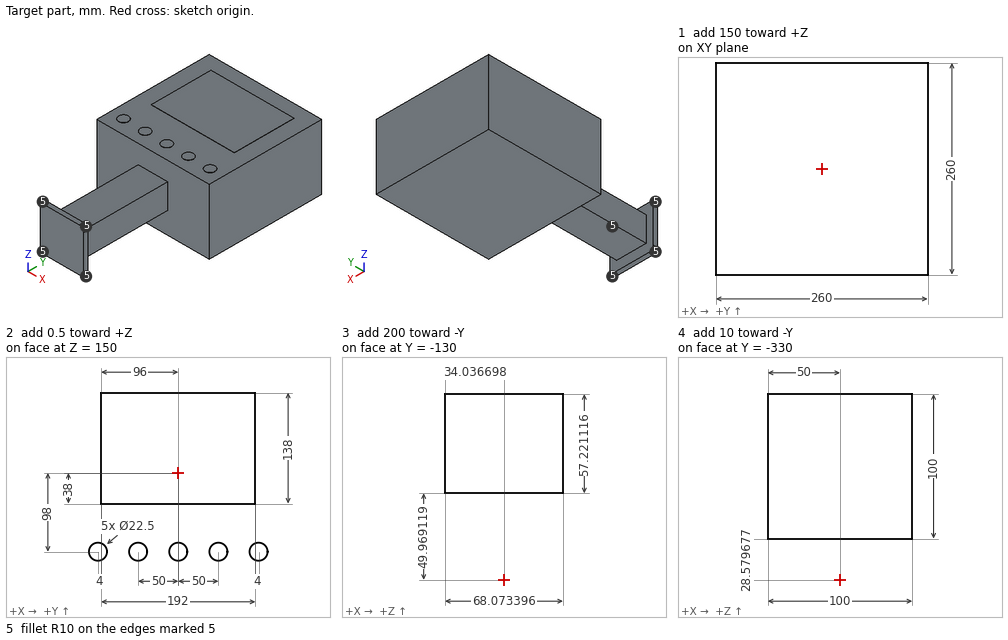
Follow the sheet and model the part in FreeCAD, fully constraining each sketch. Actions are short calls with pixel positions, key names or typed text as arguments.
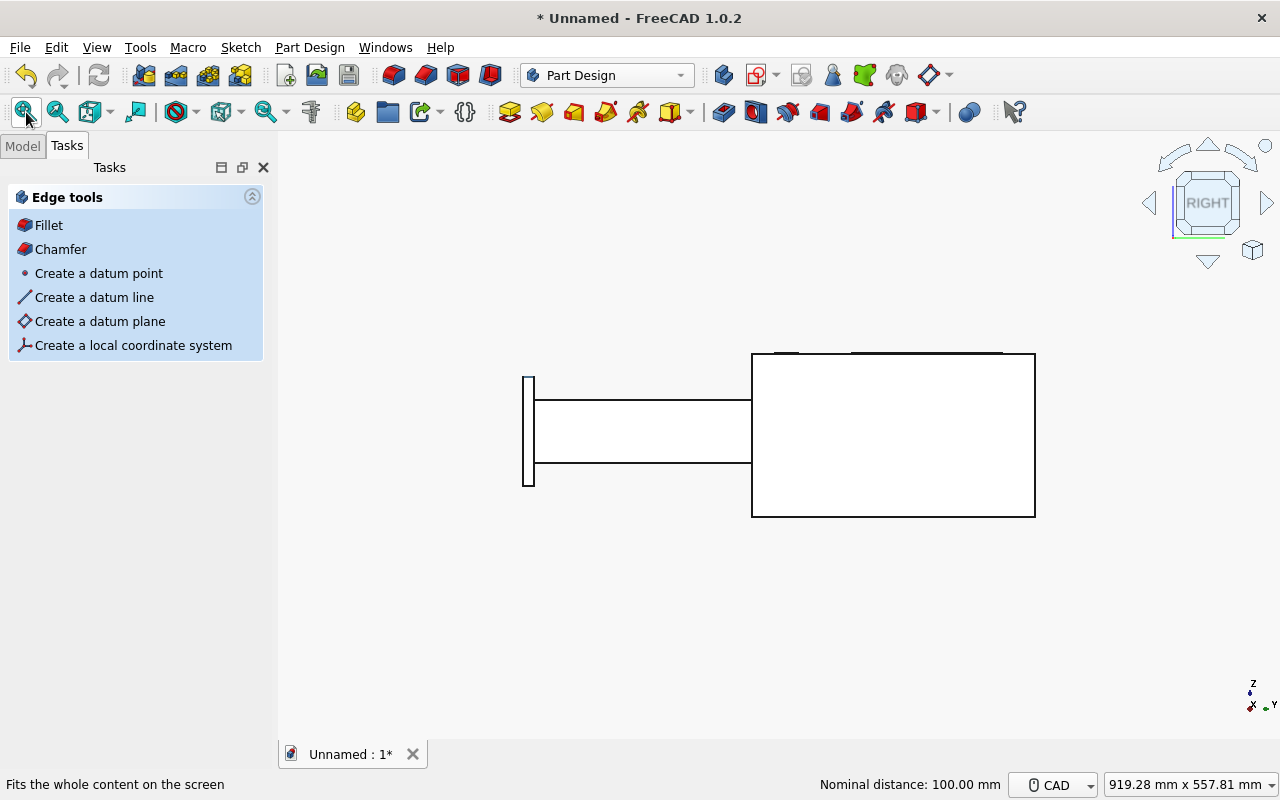
scroll(528, 485, up, 7)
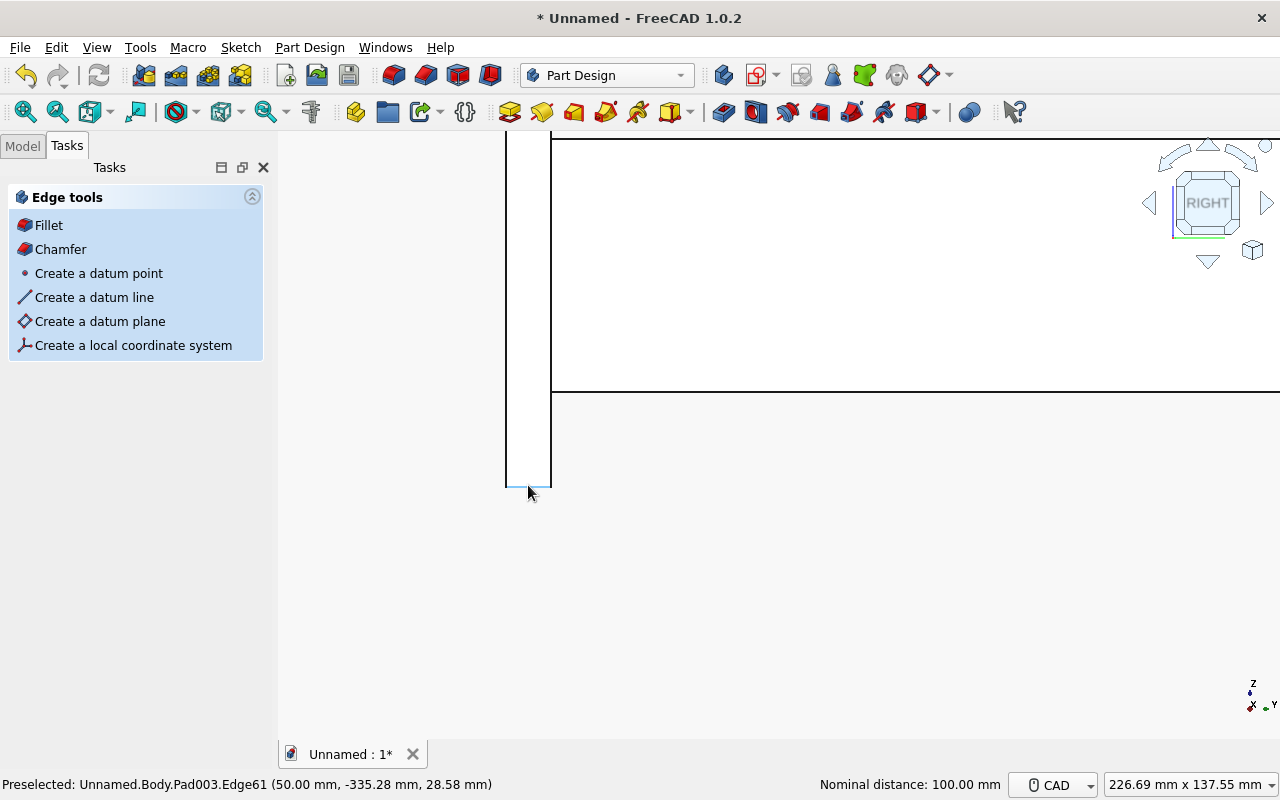
click(528, 486, ctrl)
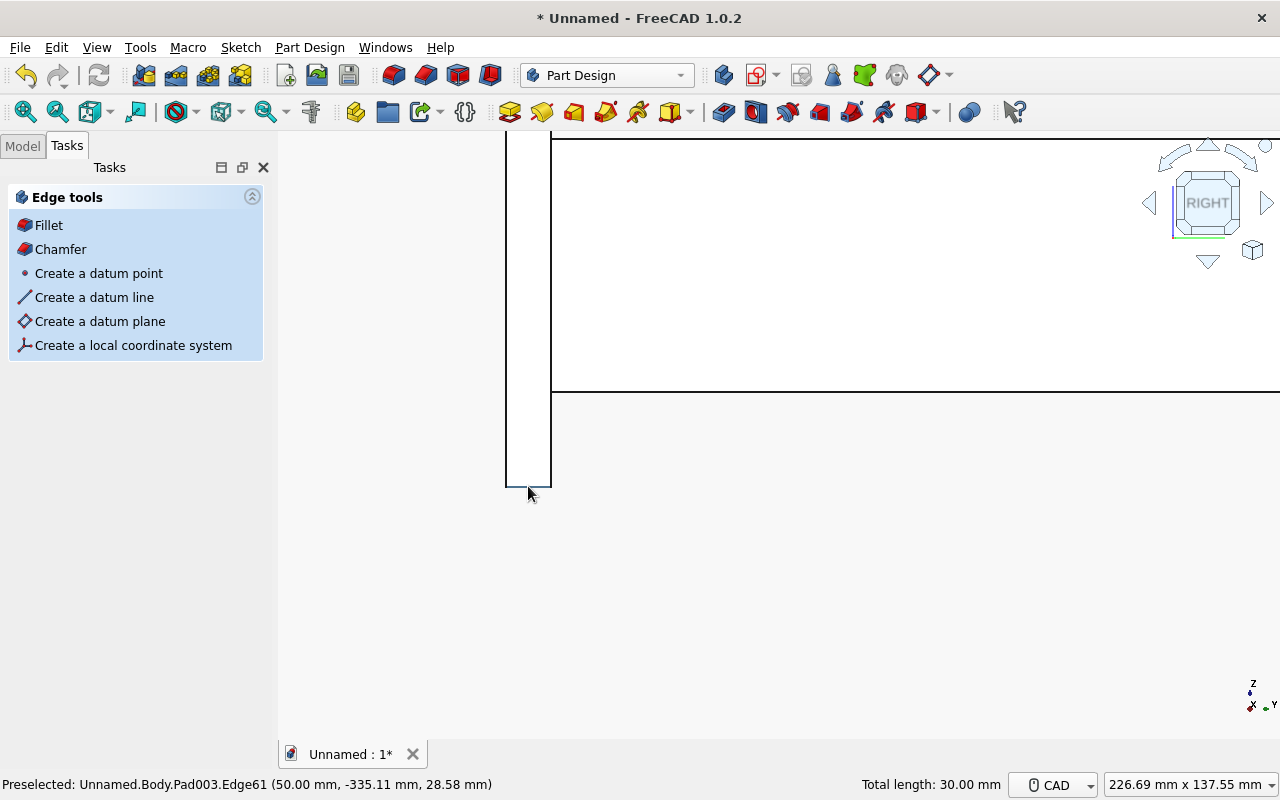
key(v)
key(f)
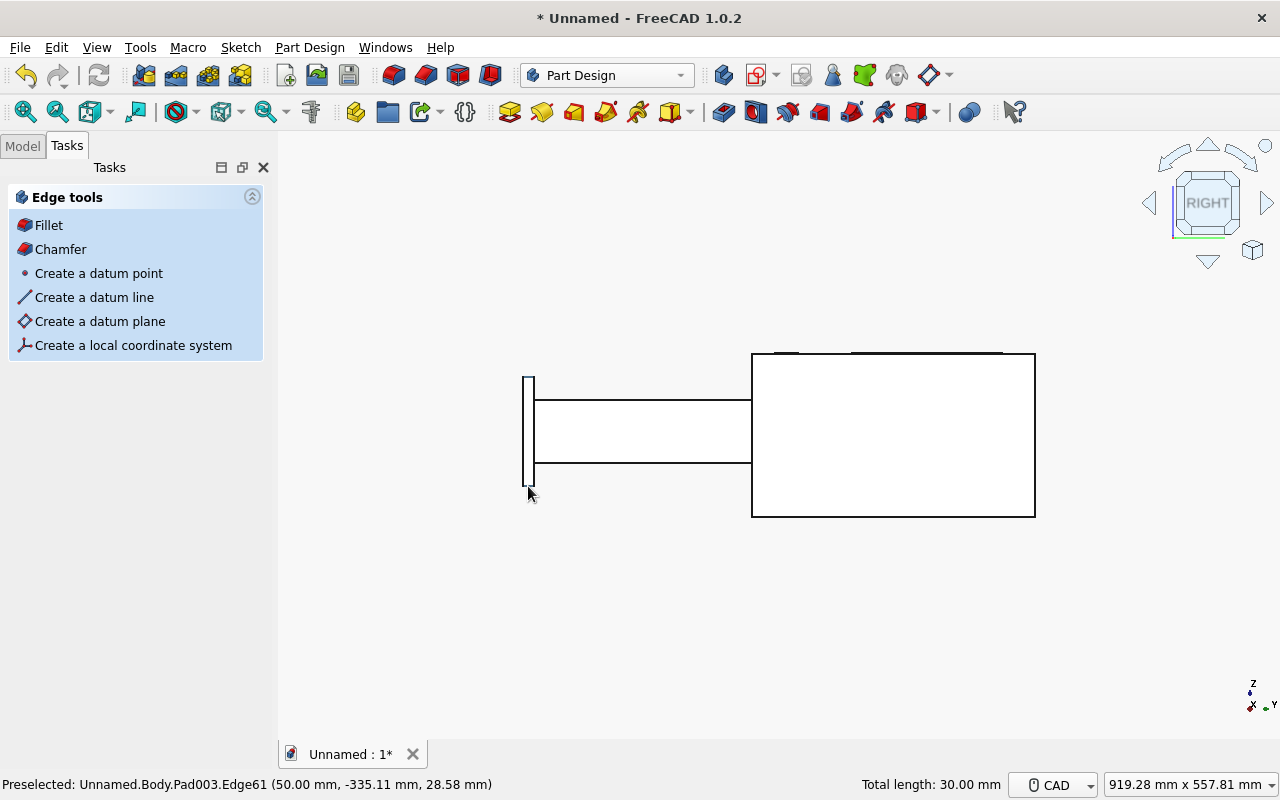
key(5)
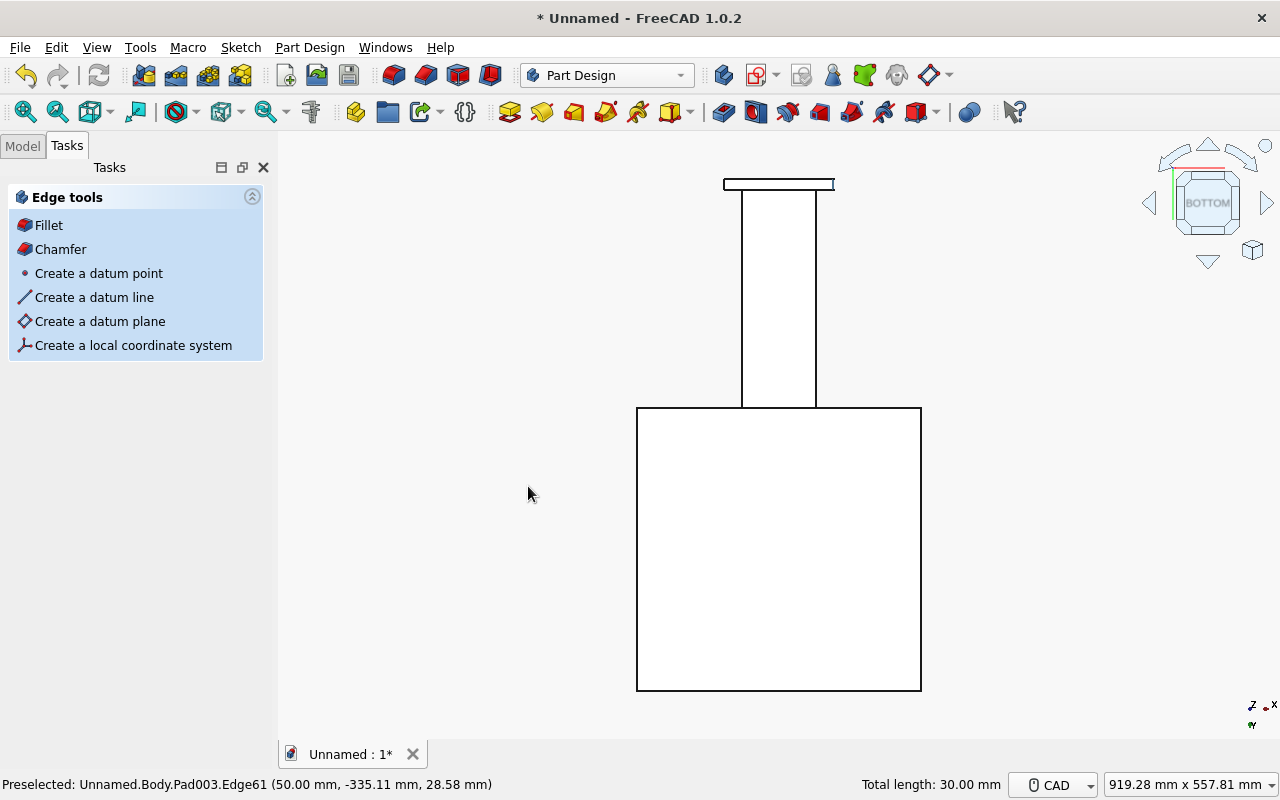
scroll(725, 183, up, 7)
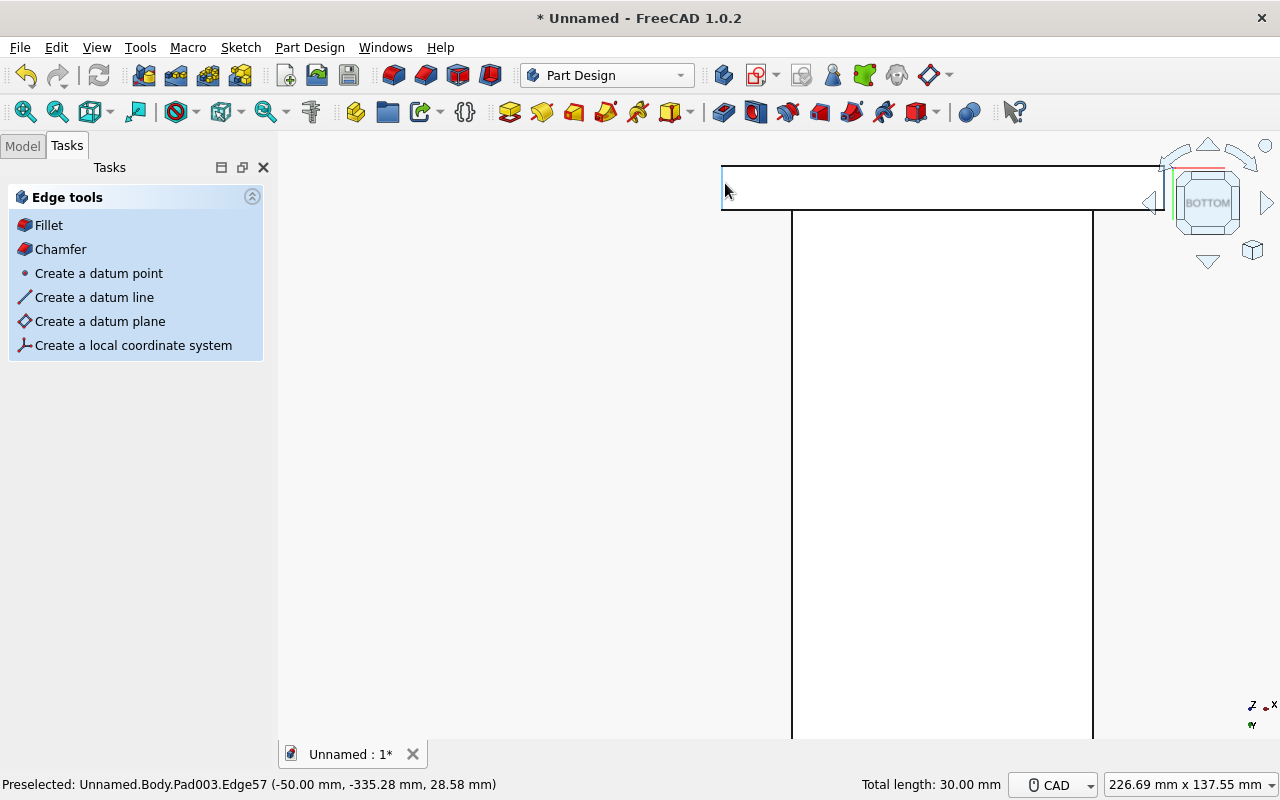
click(722, 187, ctrl)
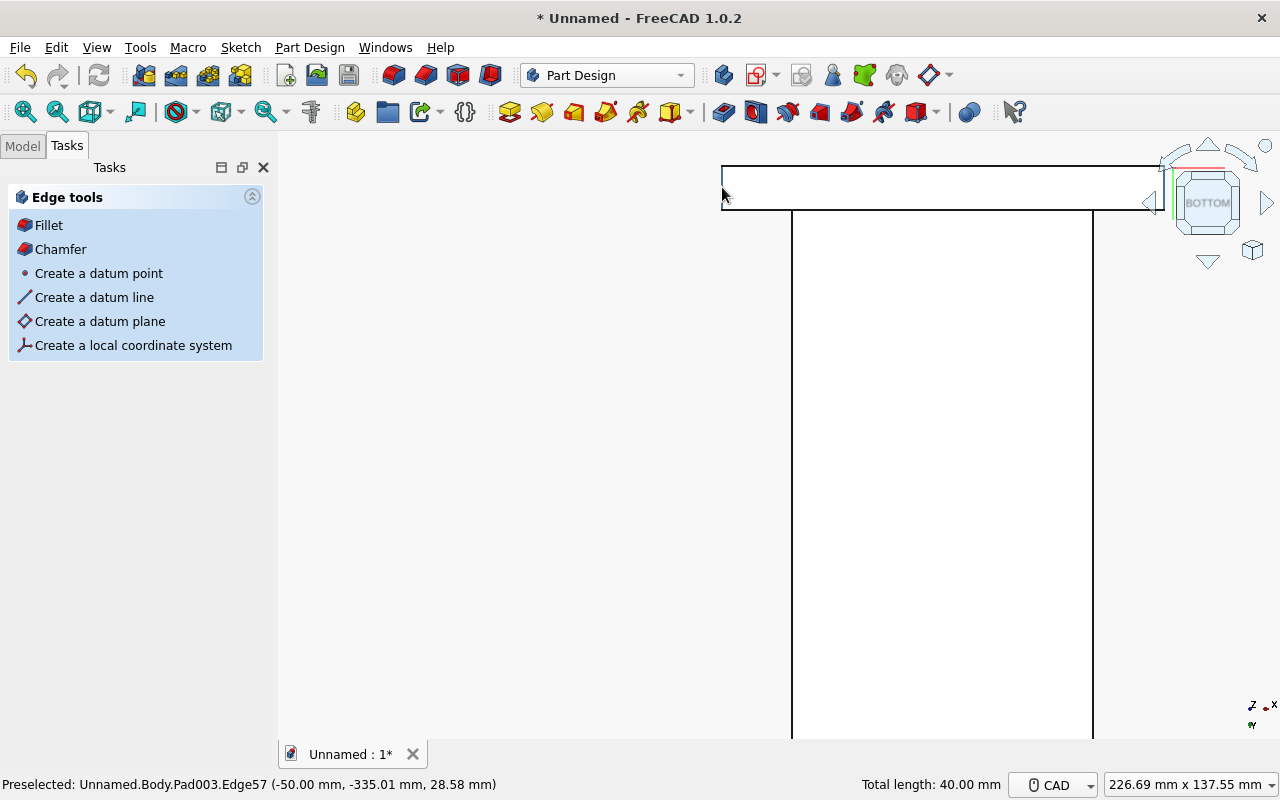
click(394, 76)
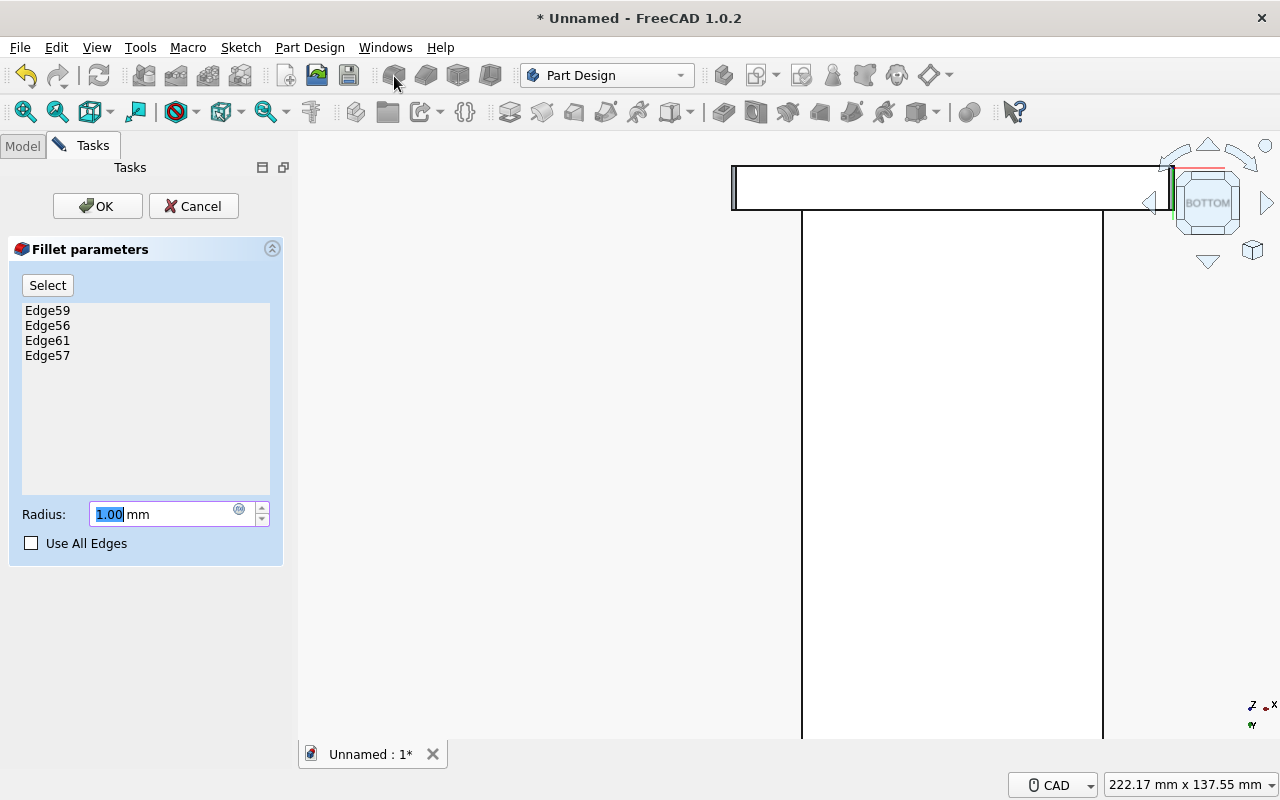
text(10)
key(Tab)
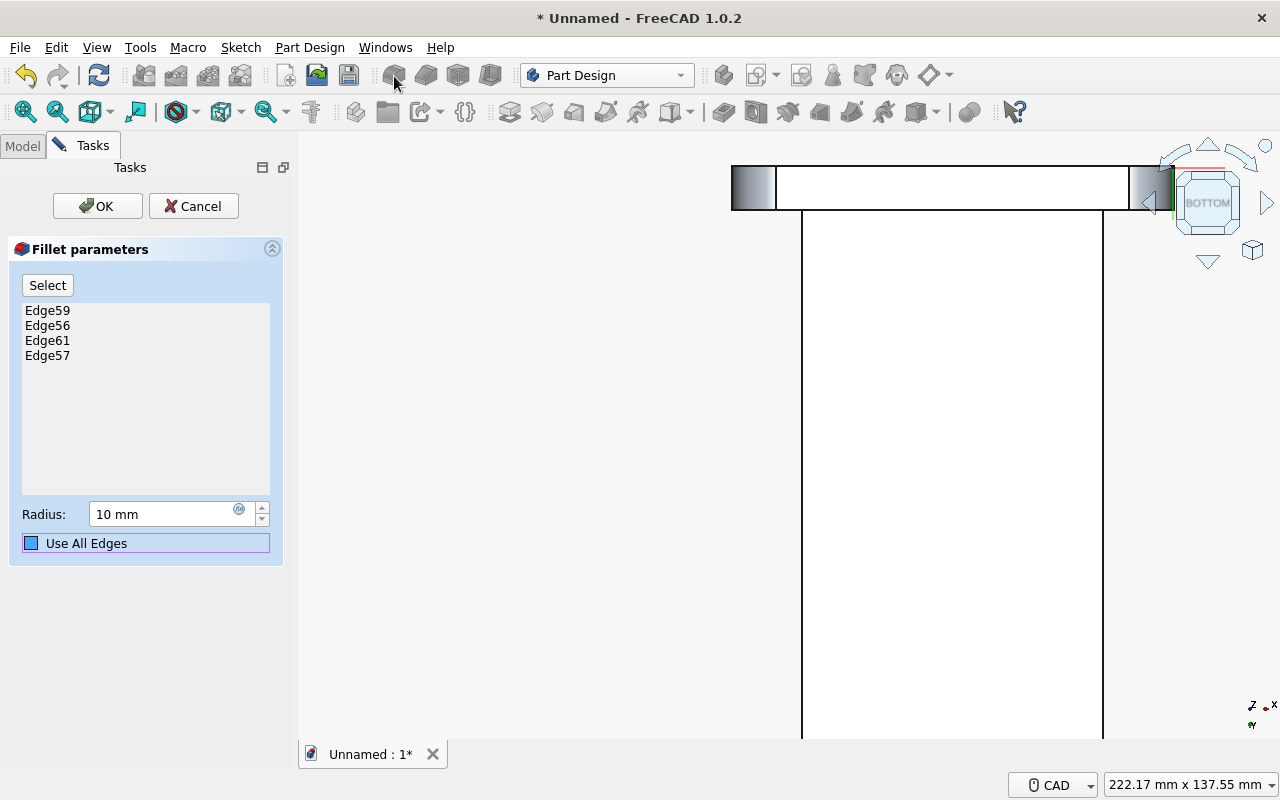
click(98, 206)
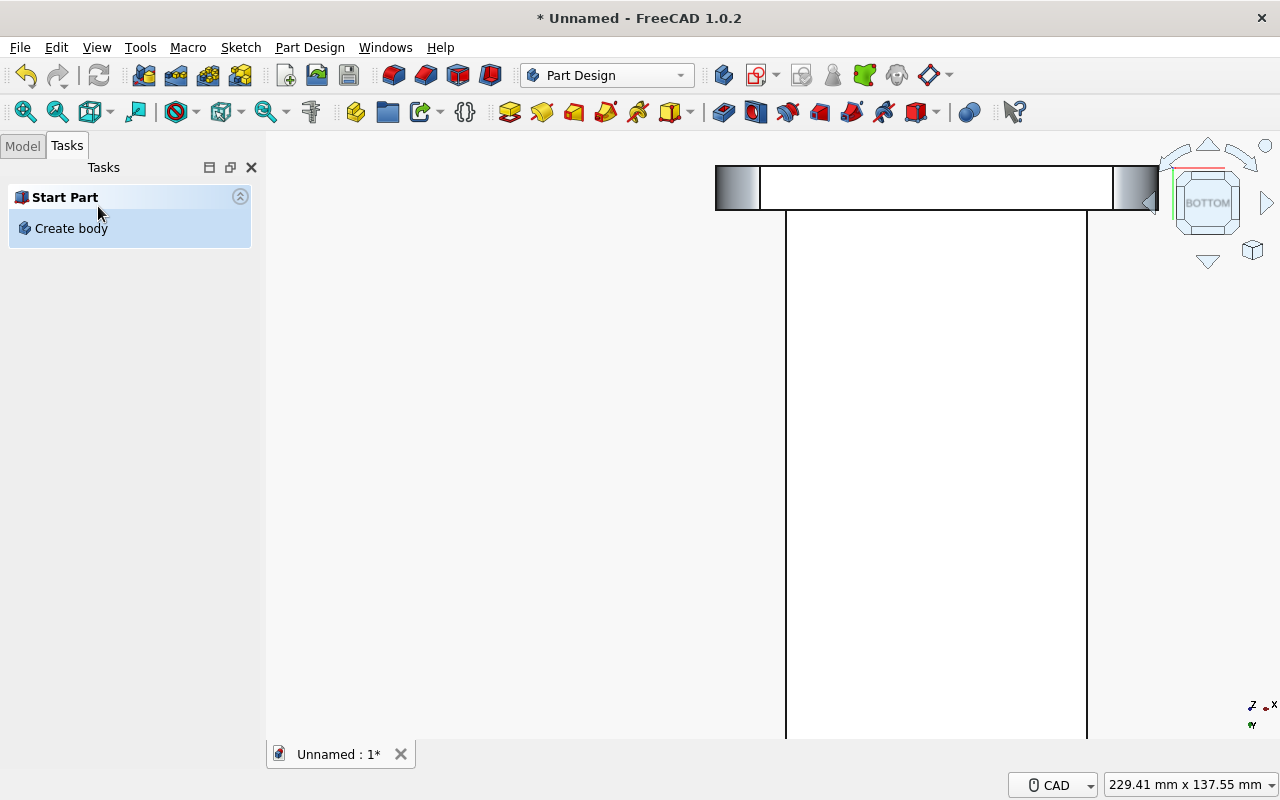
key(0)